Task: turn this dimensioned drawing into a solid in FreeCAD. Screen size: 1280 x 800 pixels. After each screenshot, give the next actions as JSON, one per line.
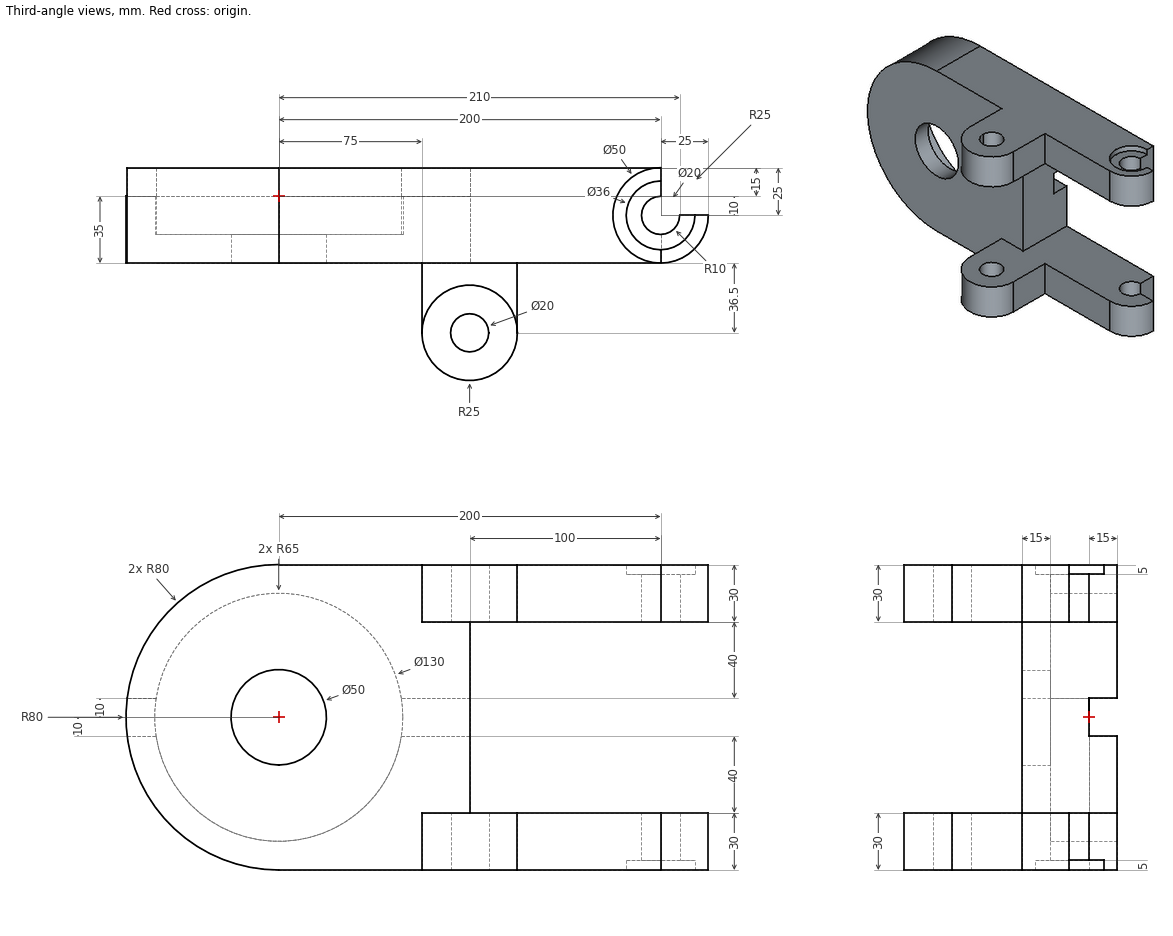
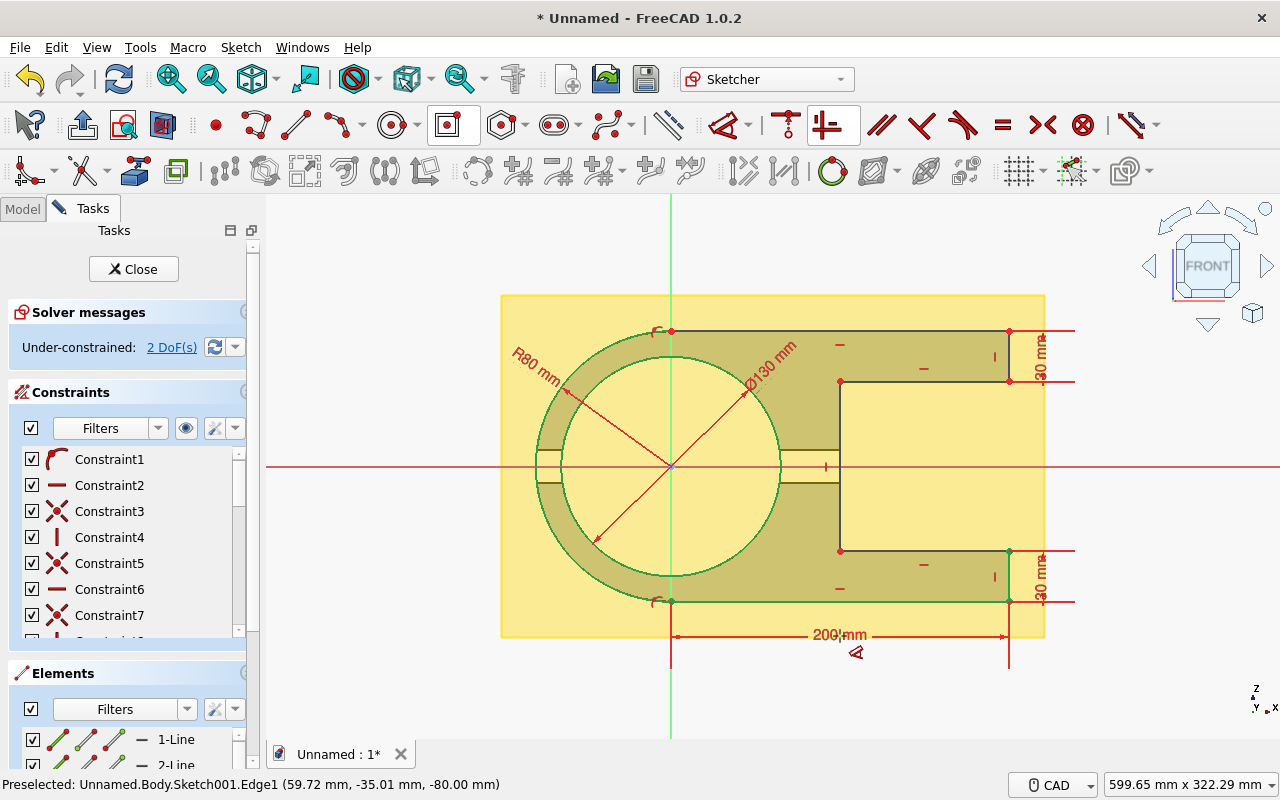
{"action": "left_click", "coordinate": [958, 551]}
{"action": "left_click", "coordinate": [925, 585]}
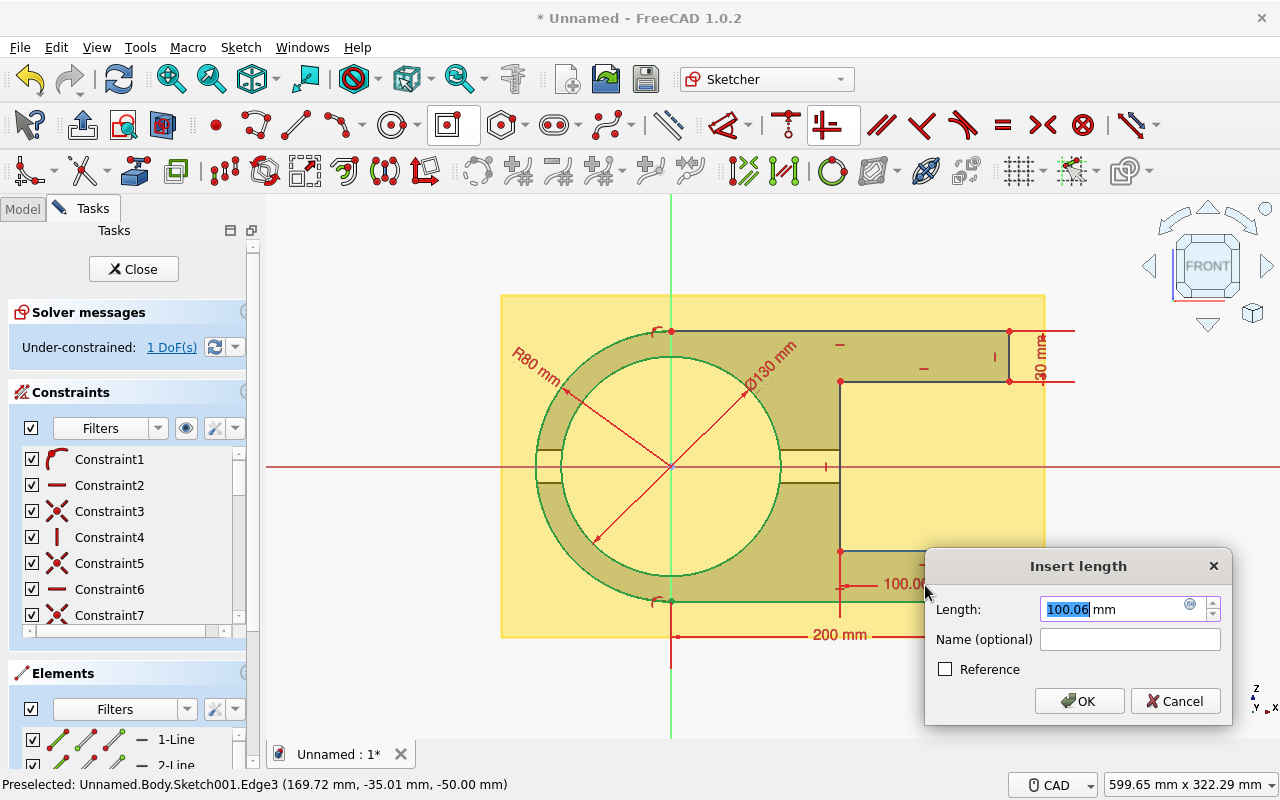
{"action": "type", "text": "100"}
{"action": "key", "text": "Return"}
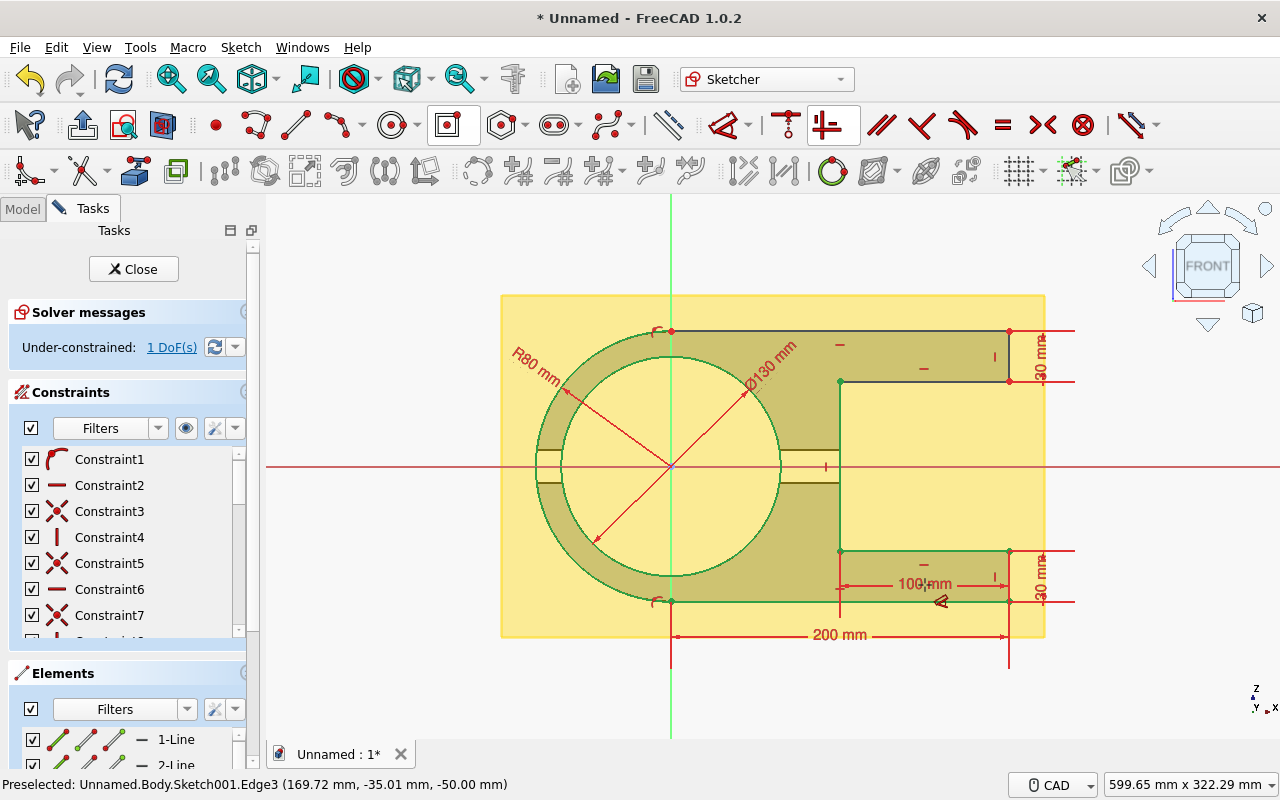
{"action": "left_click", "coordinate": [891, 382]}
{"action": "left_click", "coordinate": [925, 348]}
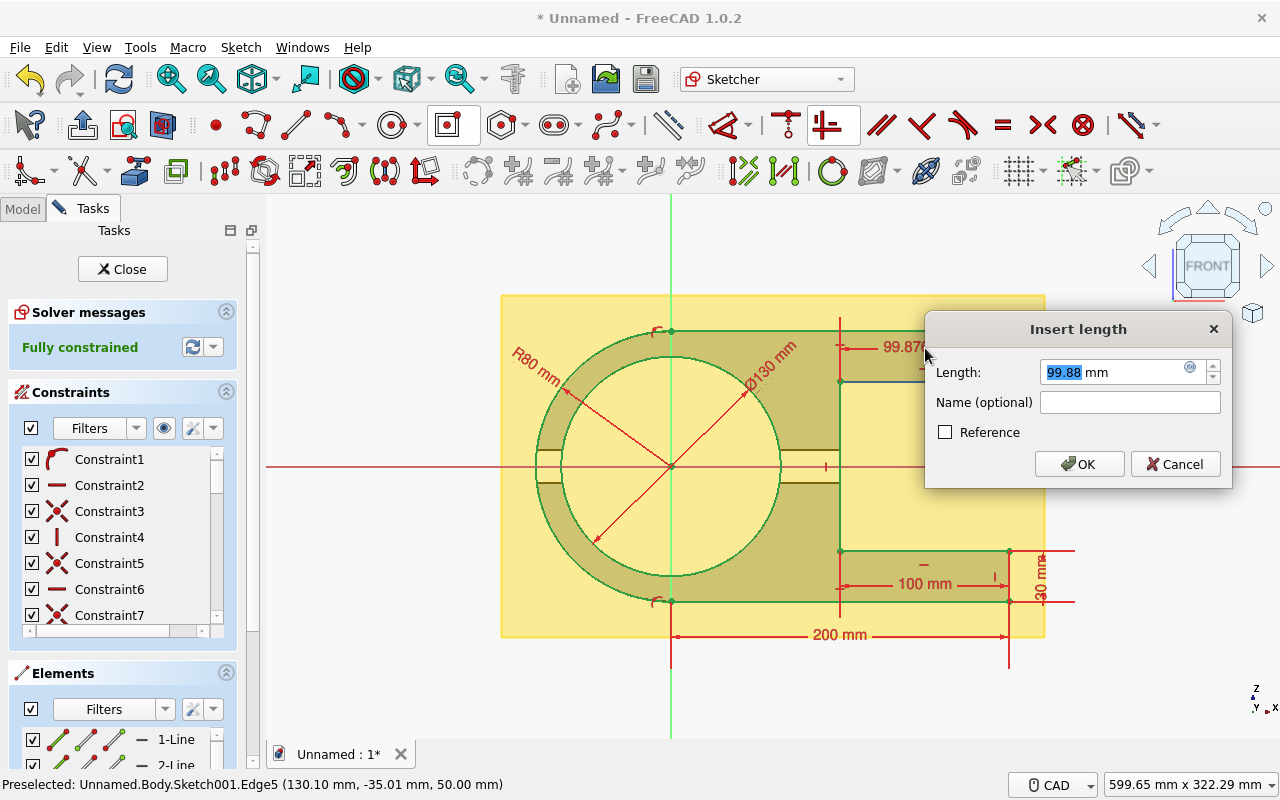
{"action": "type", "text": "100"}
{"action": "key", "text": "Return"}
{"action": "key", "text": "Escape"}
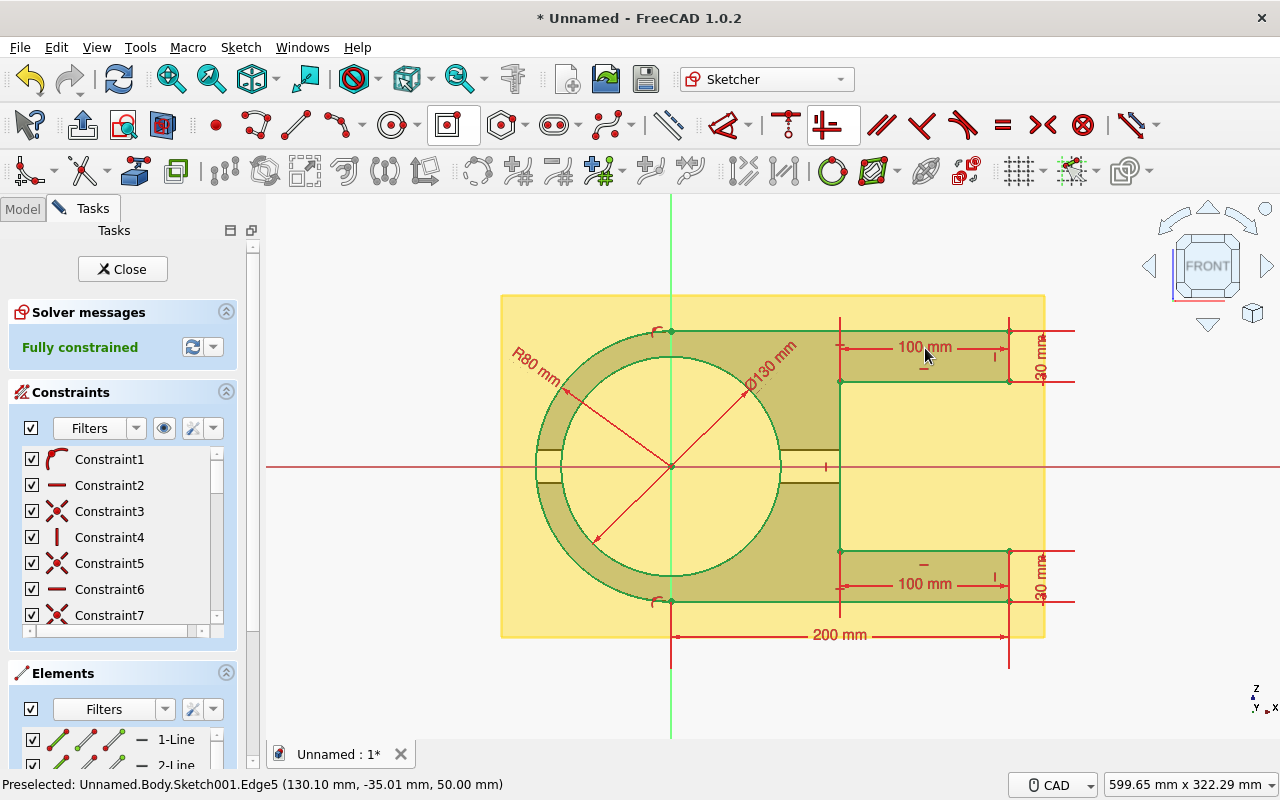
{"action": "left_click", "coordinate": [123, 269]}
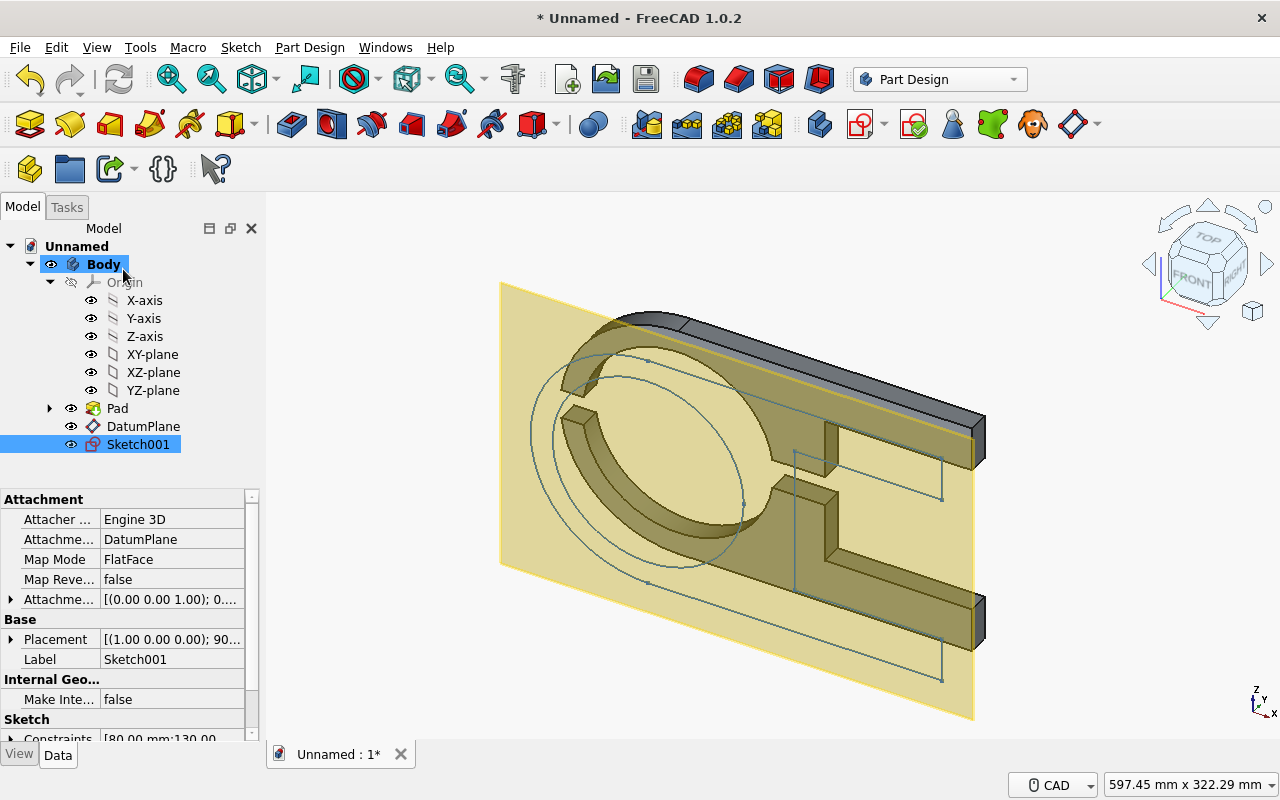
{"action": "left_click", "coordinate": [30, 124]}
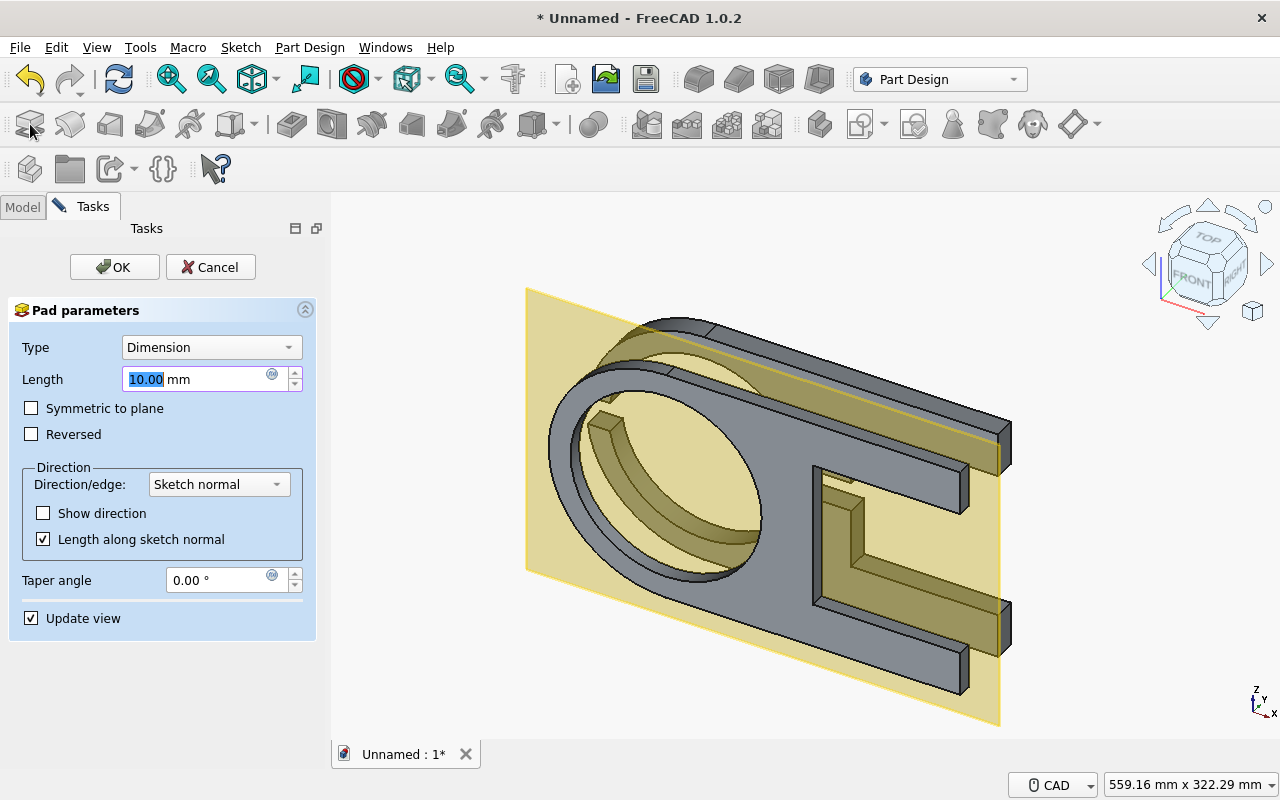
{"action": "type", "text": "35"}
{"action": "key", "text": "Tab"}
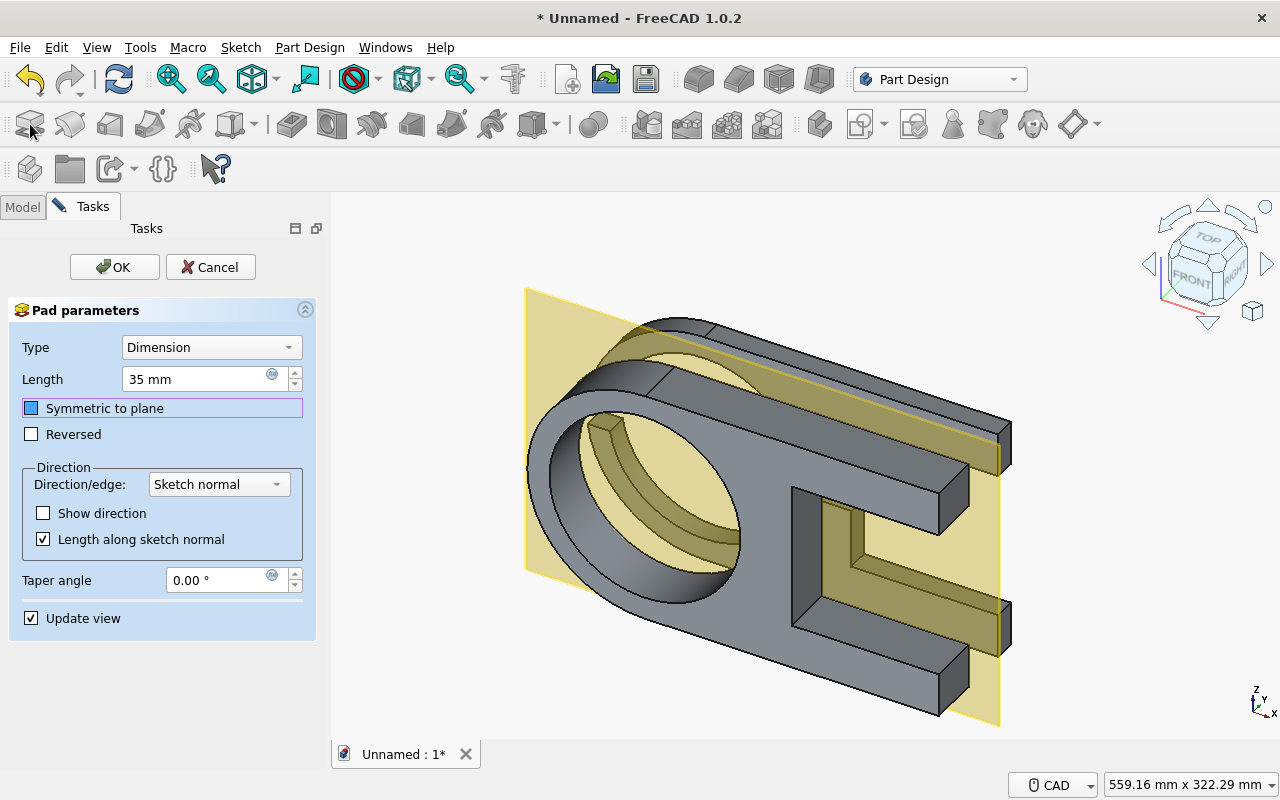
{"action": "left_click", "coordinate": [30, 434]}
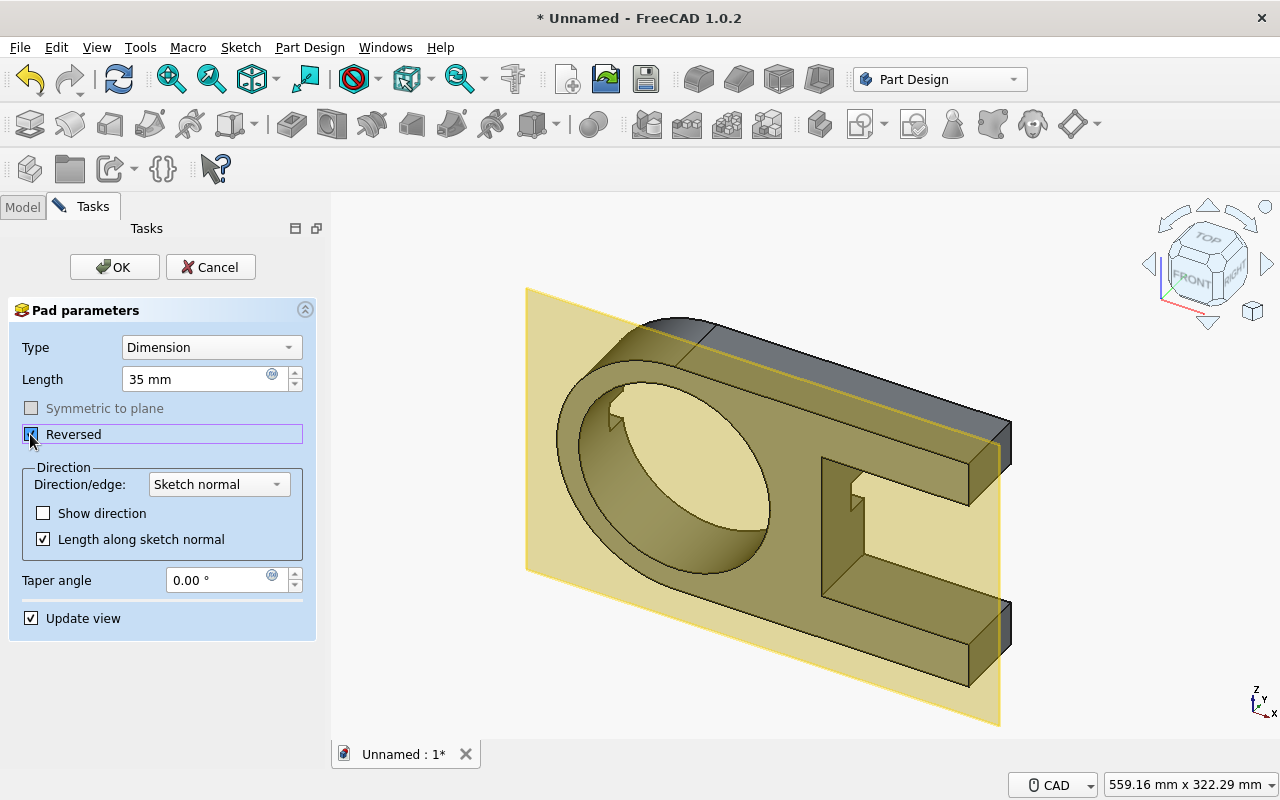
{"action": "left_click", "coordinate": [115, 267]}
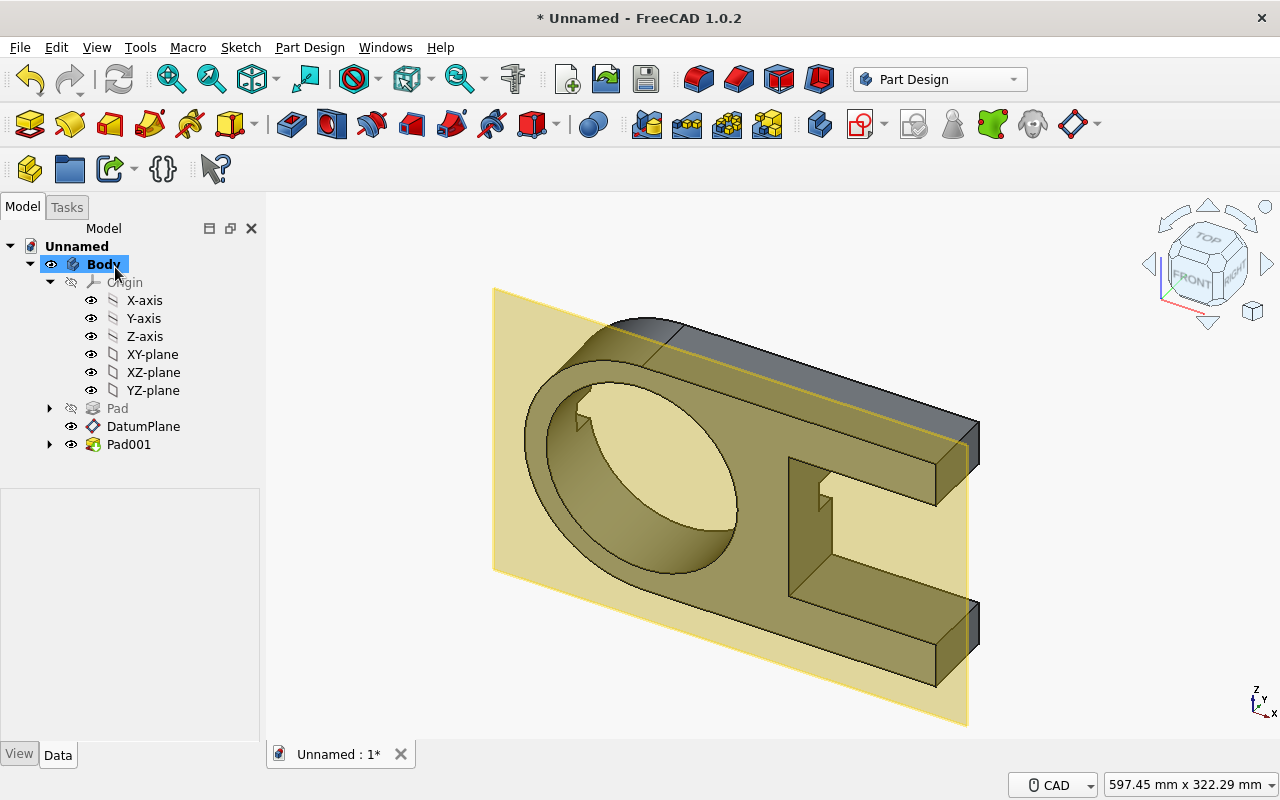
{"action": "left_click", "coordinate": [116, 426]}
{"action": "key", "text": "space"}